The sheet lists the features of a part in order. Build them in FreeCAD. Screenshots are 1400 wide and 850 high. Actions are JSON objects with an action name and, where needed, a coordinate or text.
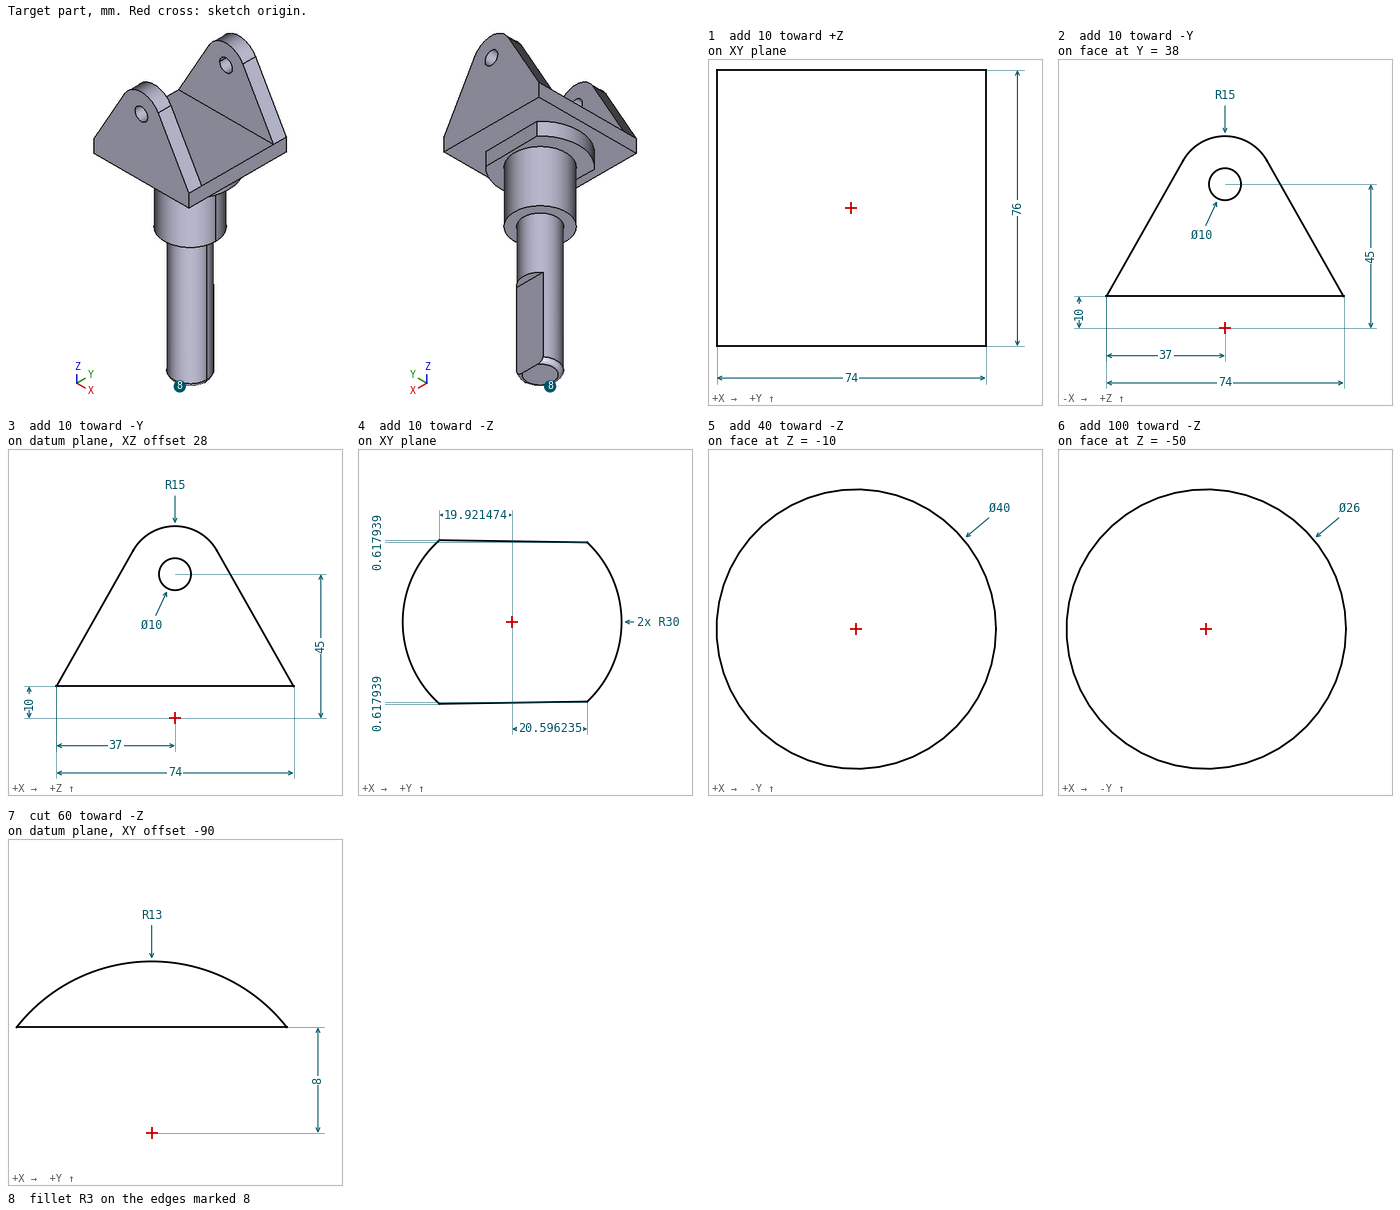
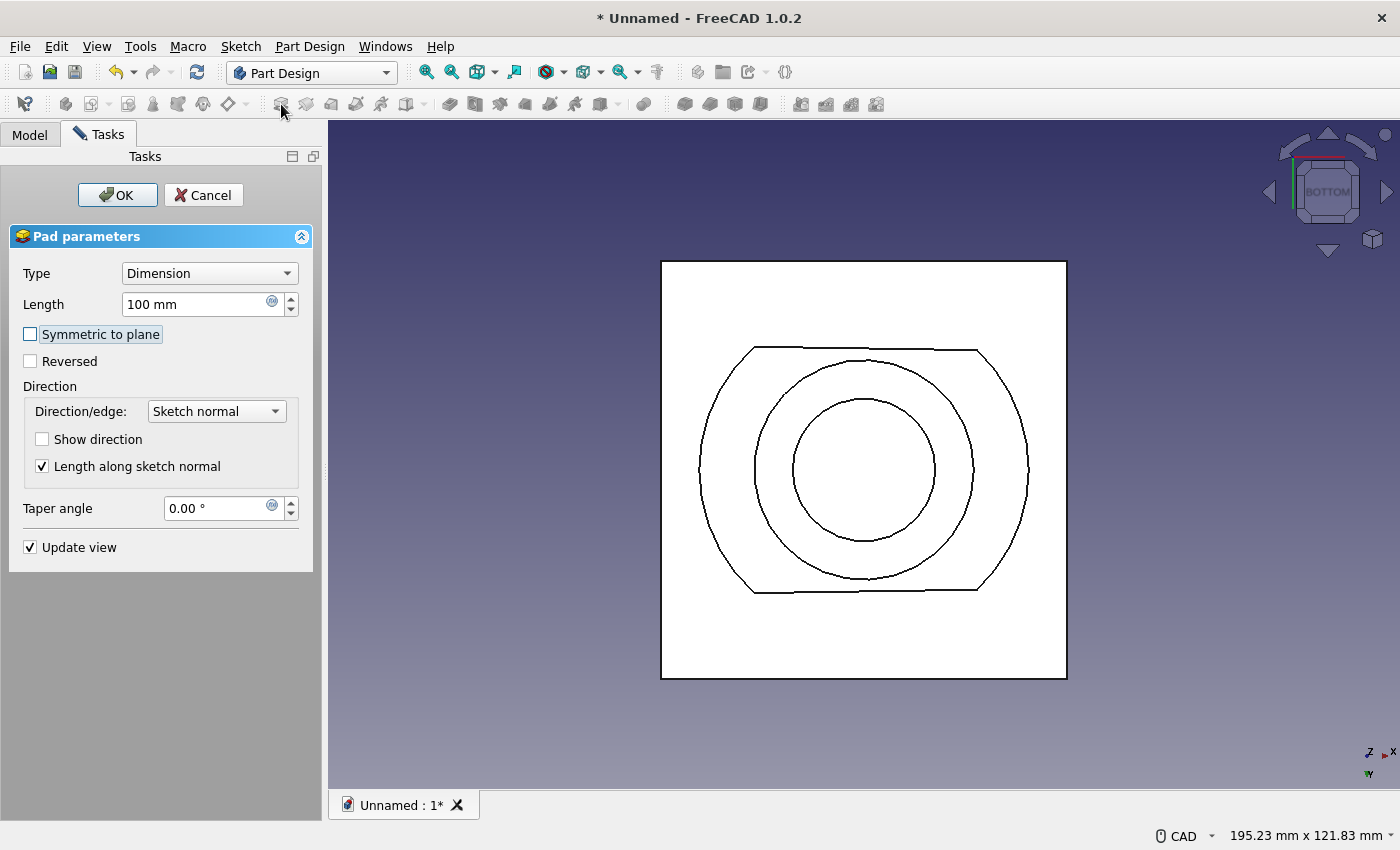
{"action": "left_click", "coordinate": [118, 195]}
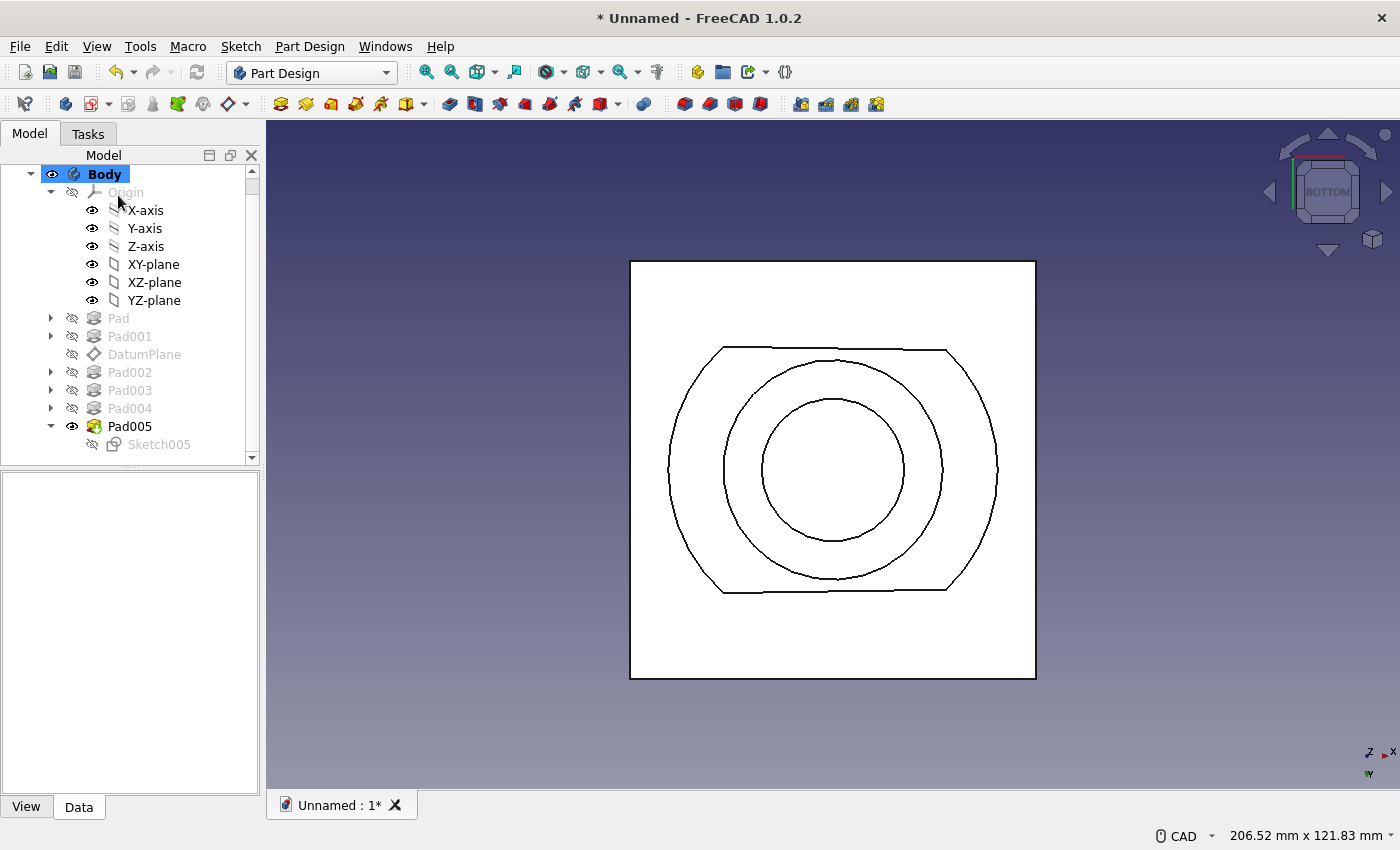
{"action": "left_click", "coordinate": [137, 264]}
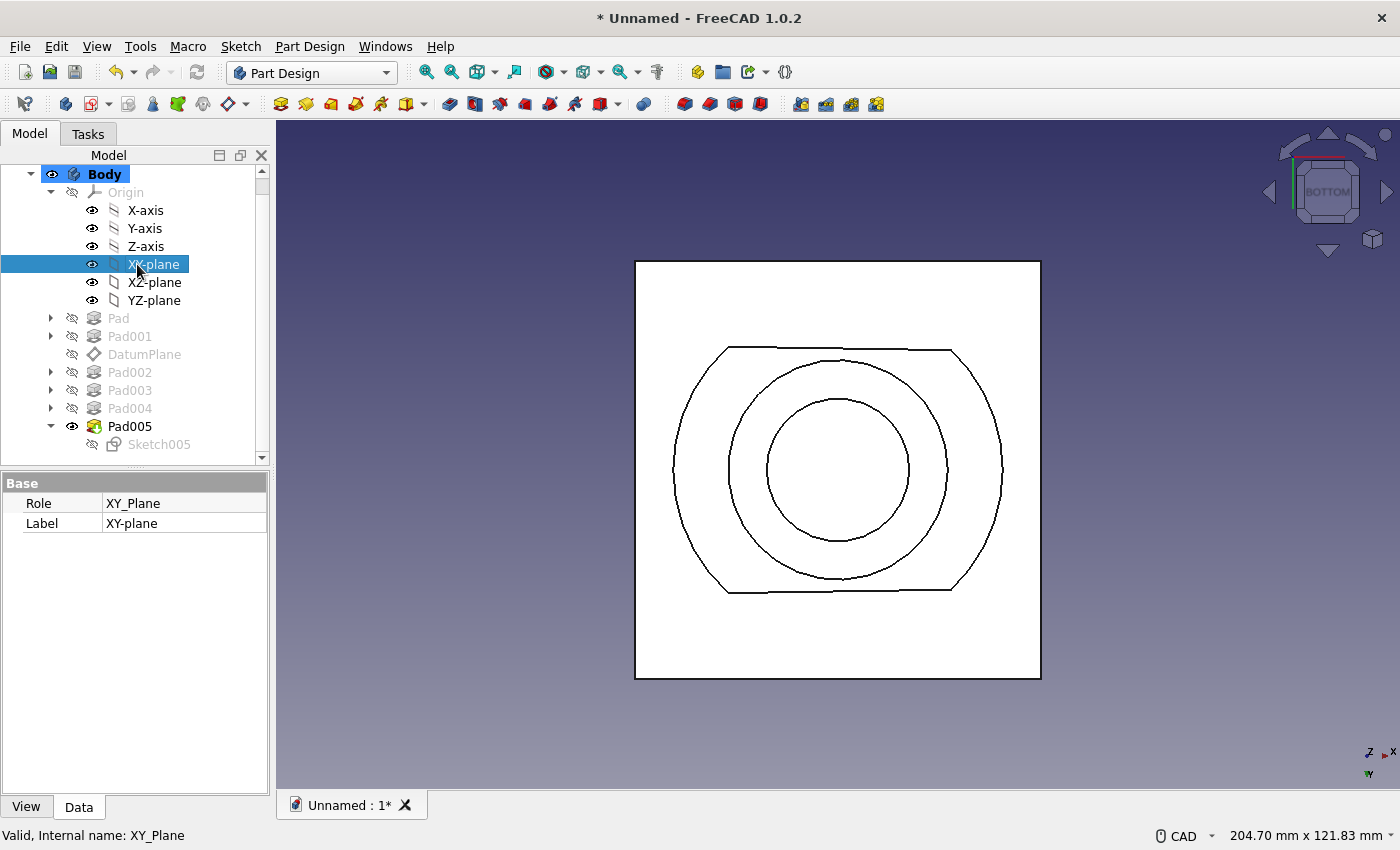
{"action": "left_click", "coordinate": [228, 104]}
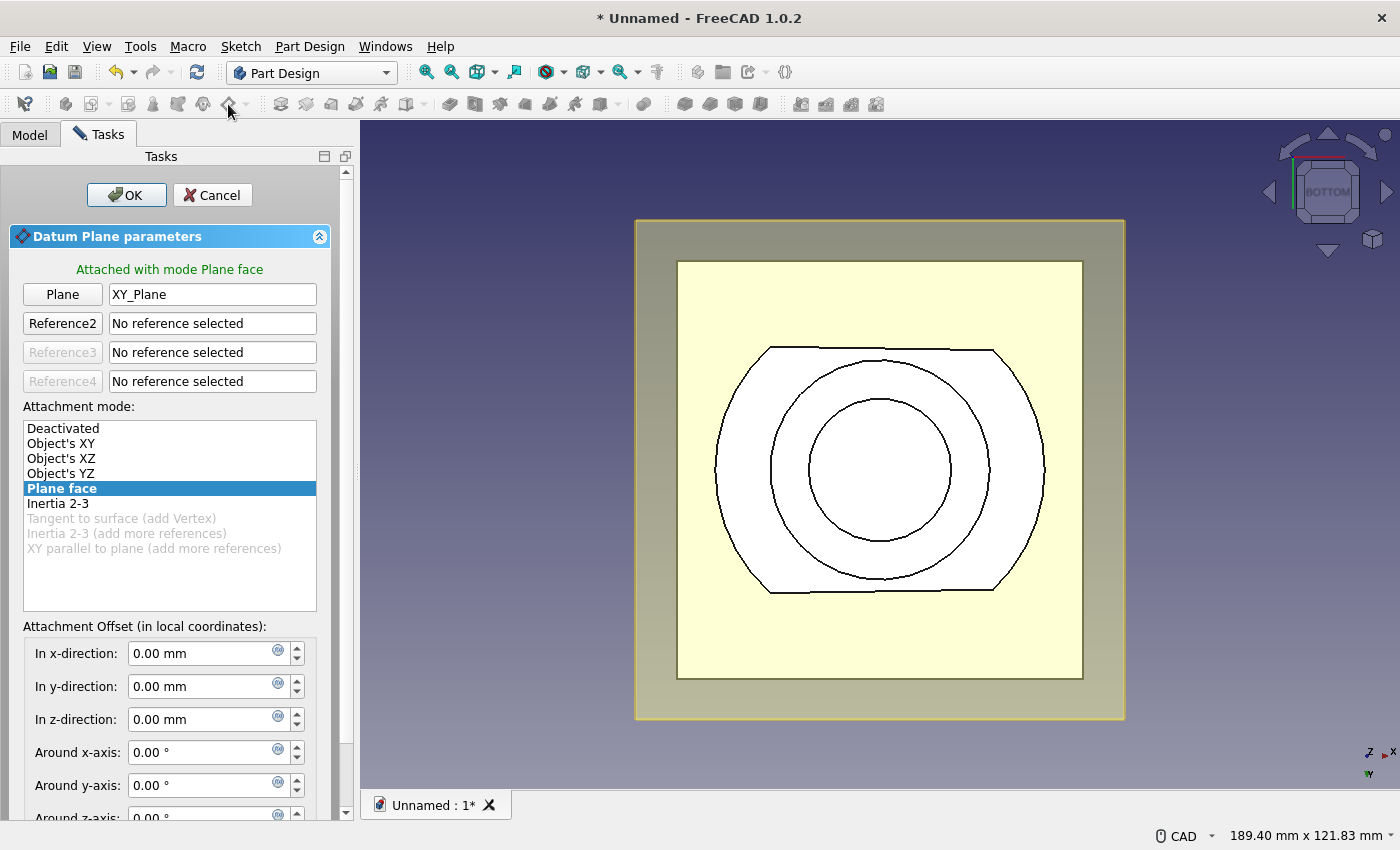
{"action": "triple_click", "coordinate": [210, 720]}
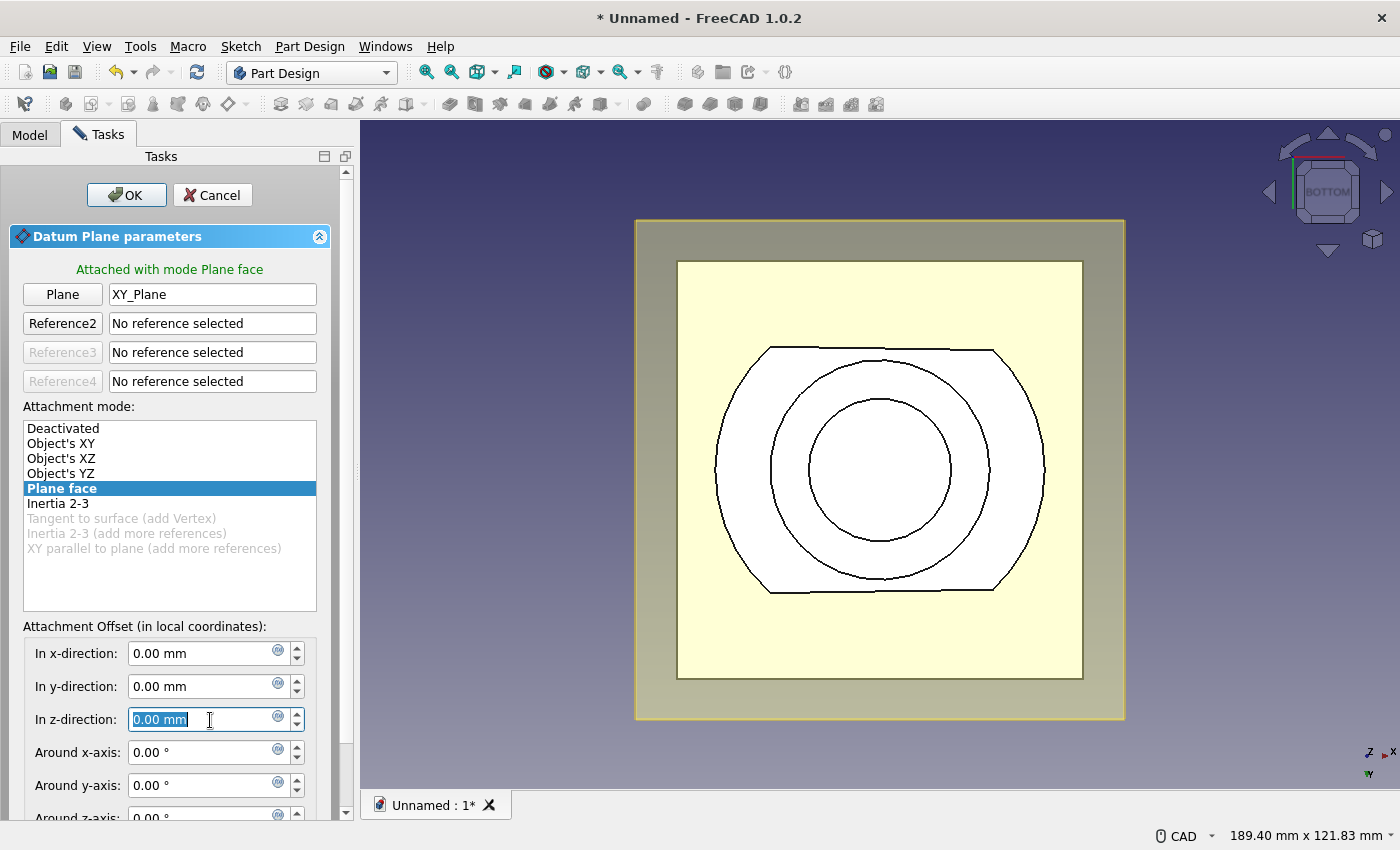
{"action": "type", "text": "-90"}
{"action": "key", "text": "Tab"}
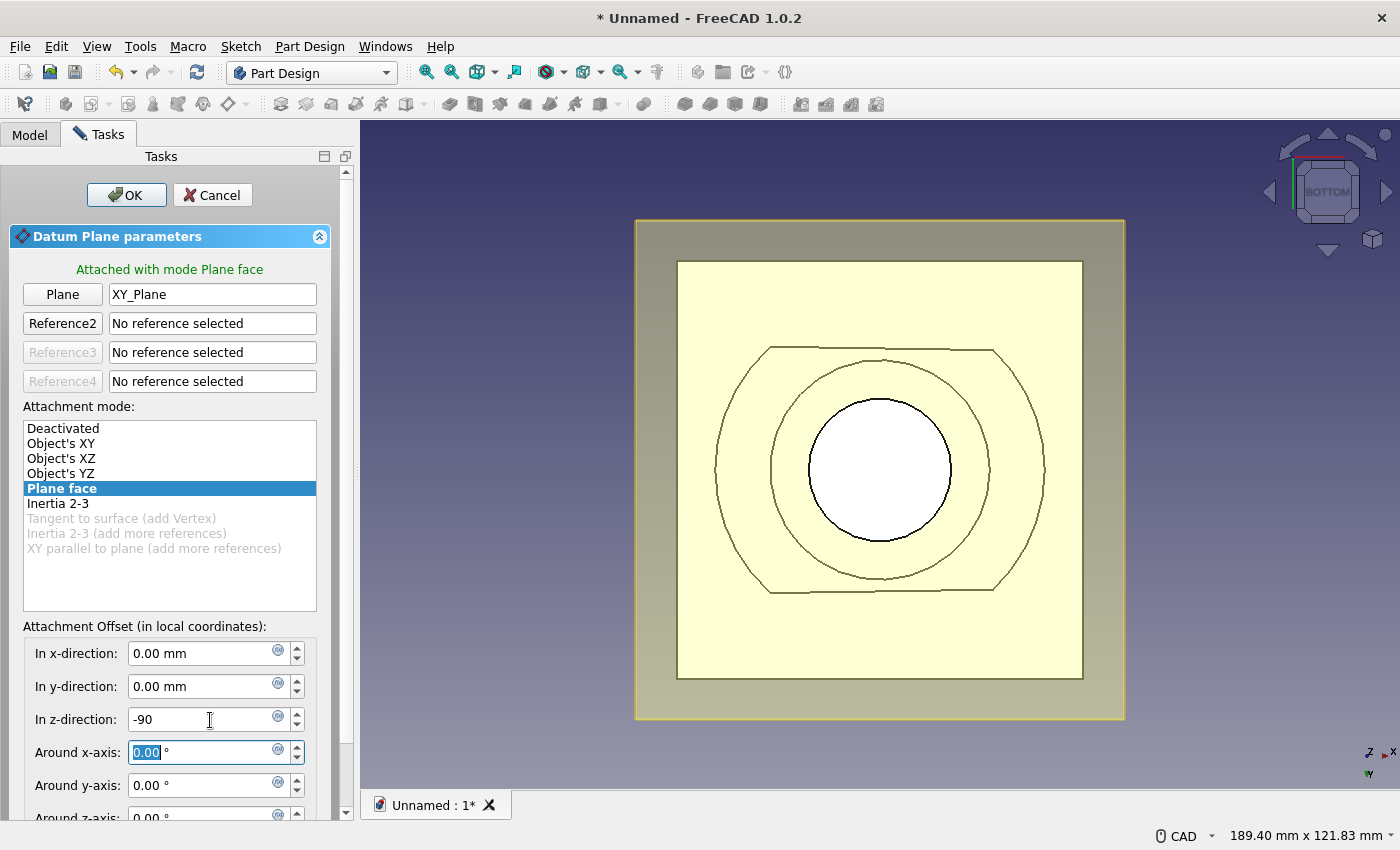
{"action": "left_click", "coordinate": [127, 195]}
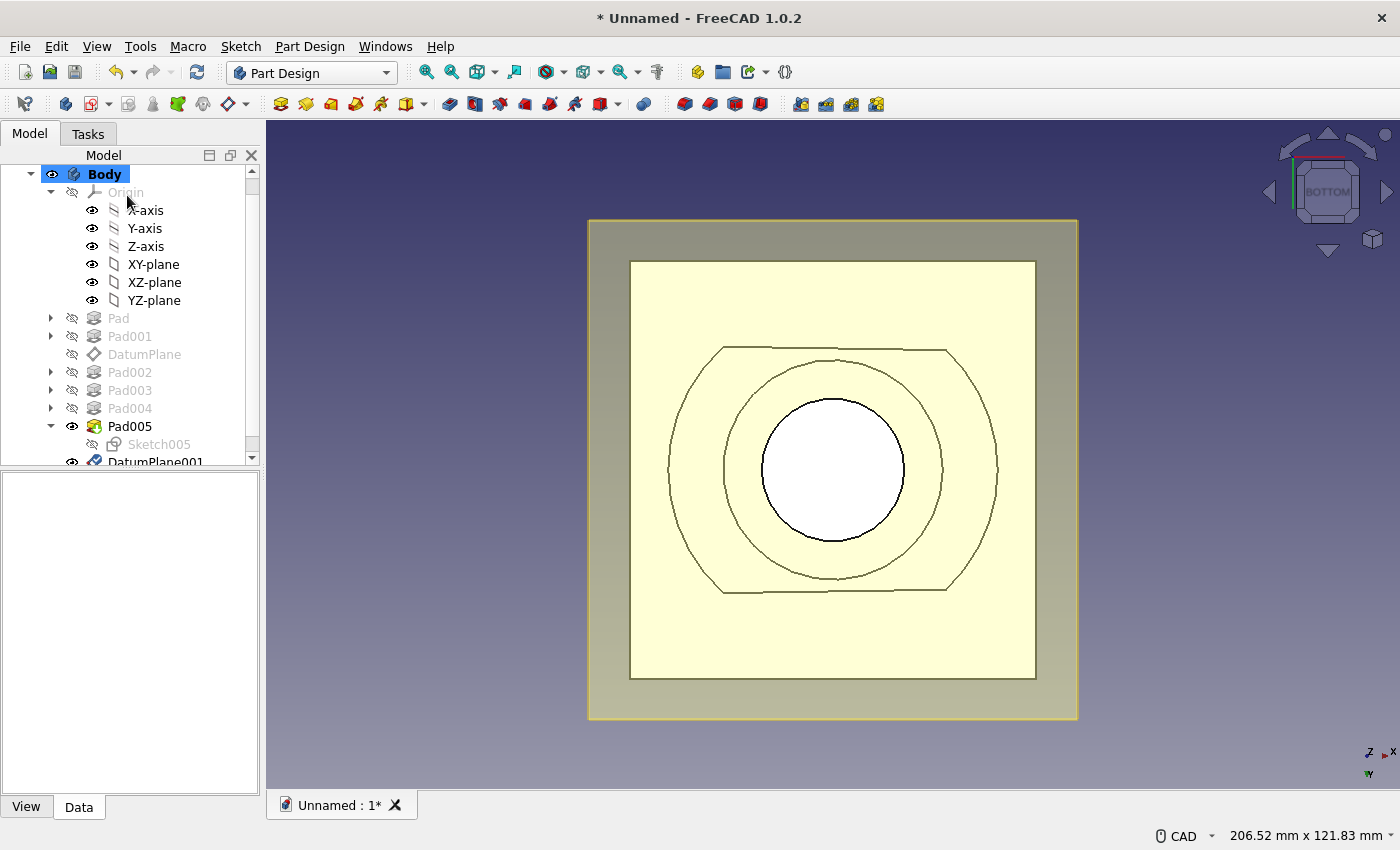
{"action": "left_click", "coordinate": [117, 462]}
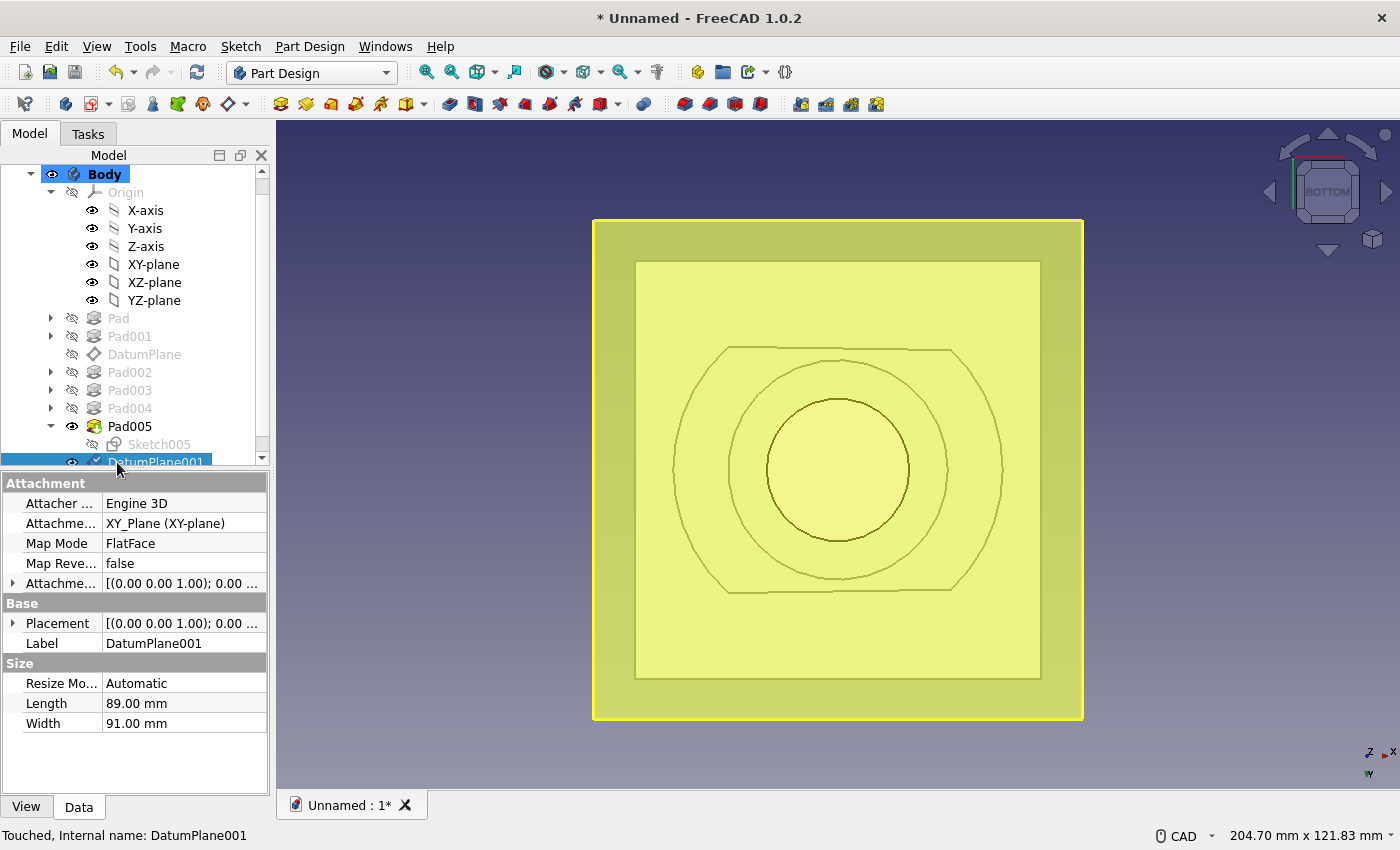
{"action": "left_click", "coordinate": [90, 104]}